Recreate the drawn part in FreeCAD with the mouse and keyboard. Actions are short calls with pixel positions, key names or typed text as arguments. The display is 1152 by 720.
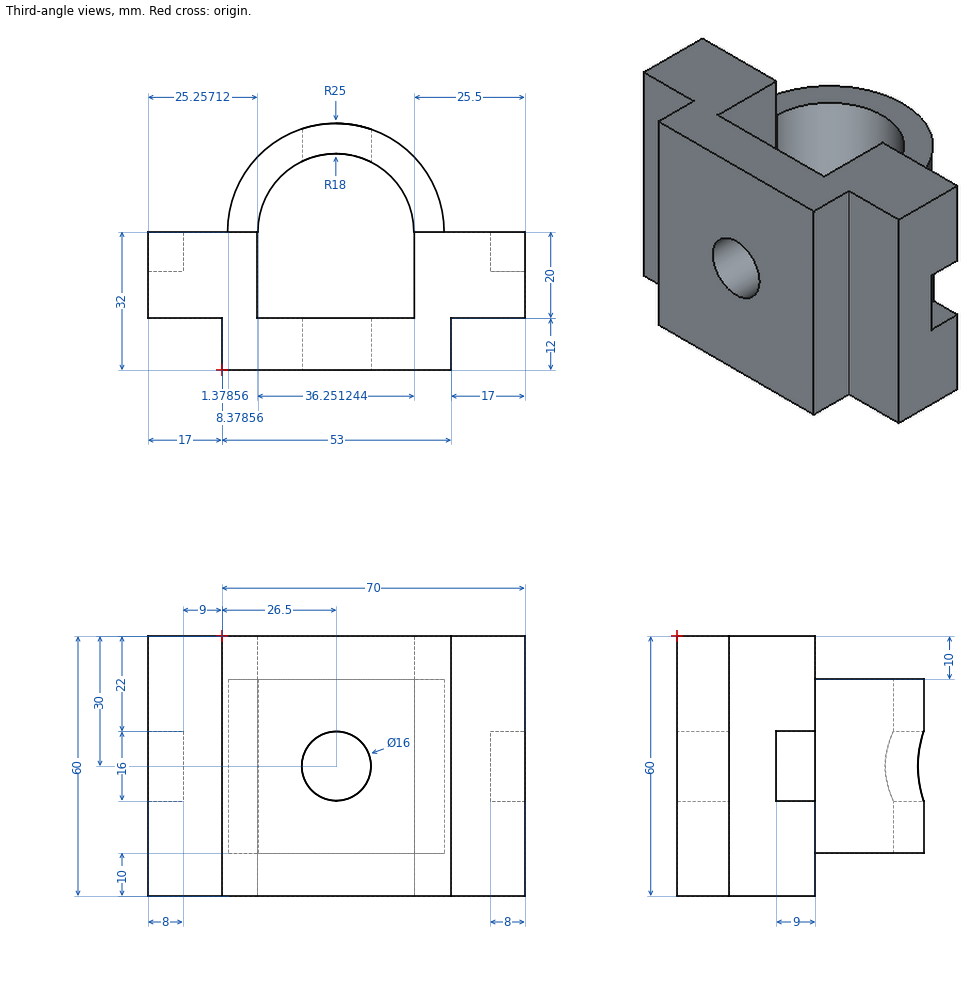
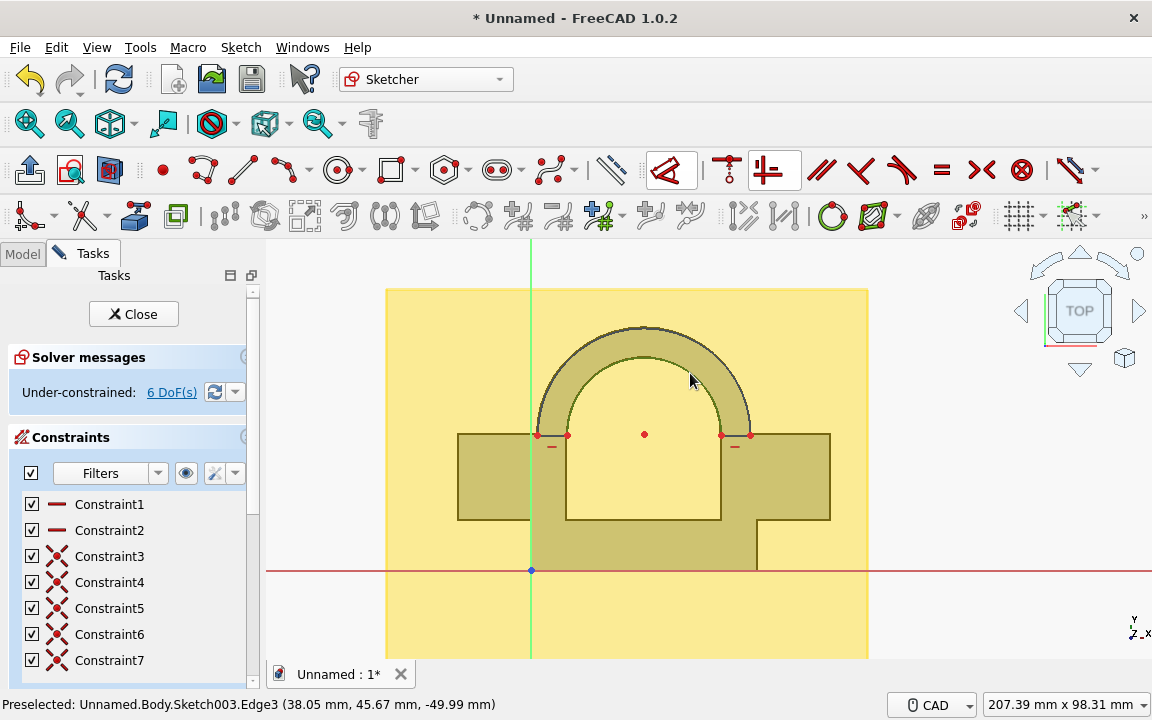
key(k)
key(r)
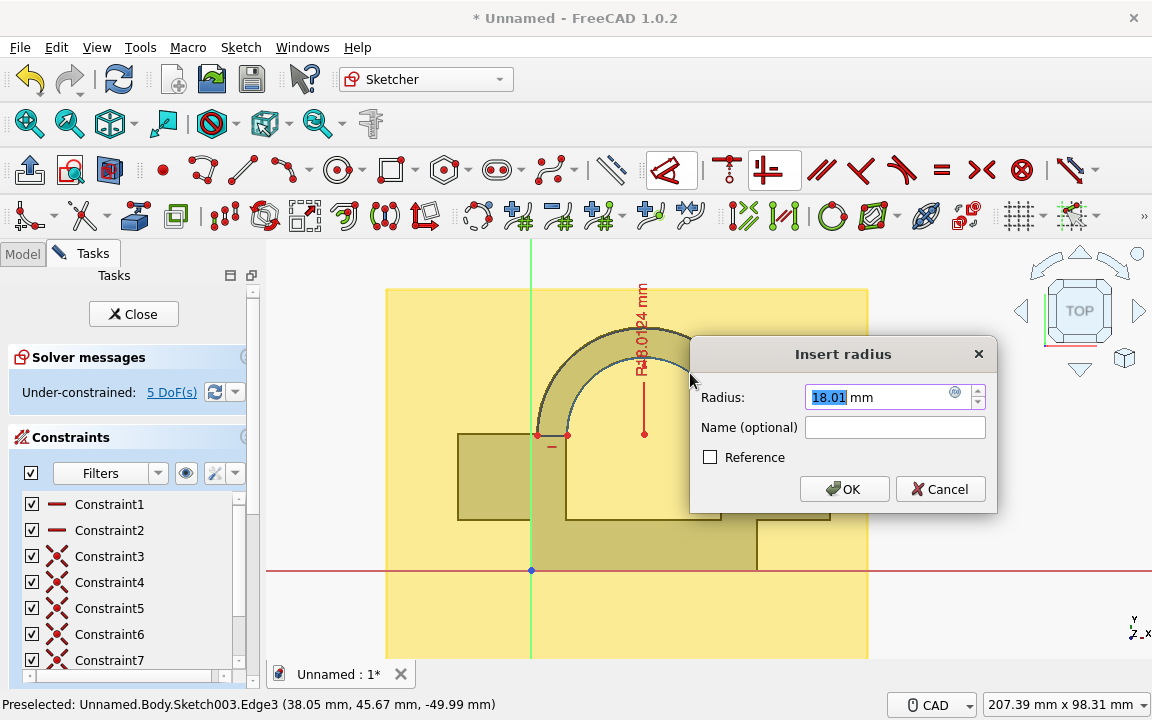
text(18)
key(Return)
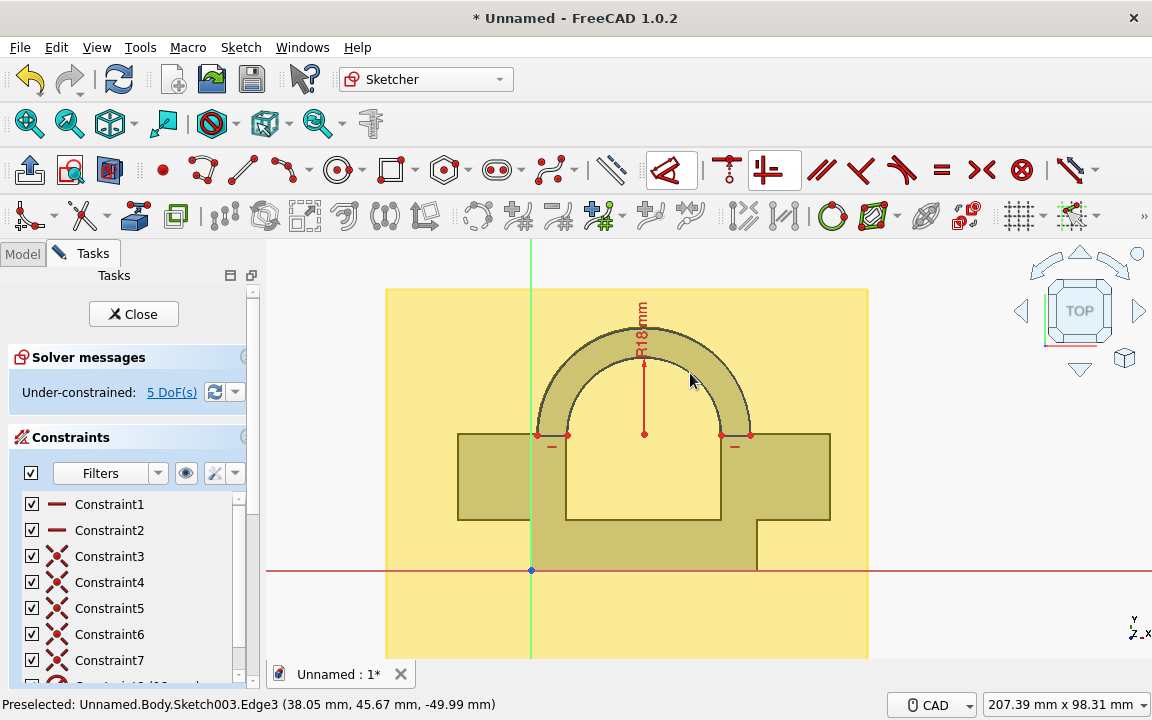
click(707, 349)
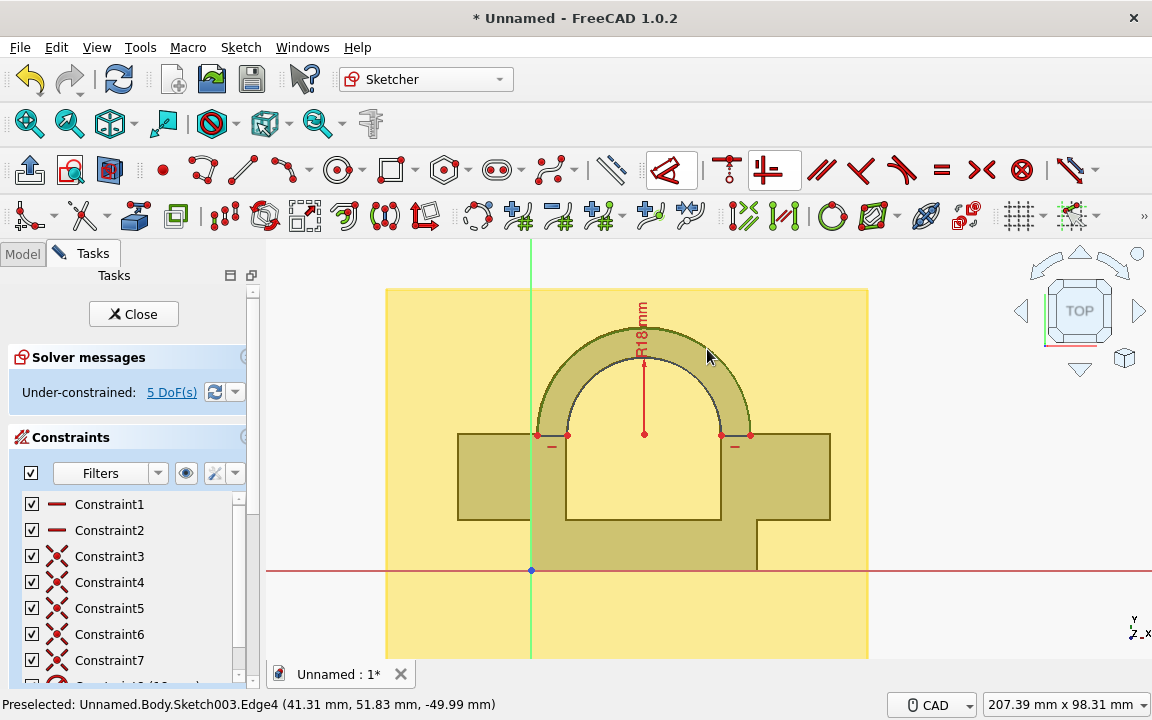
key(k)
key(r)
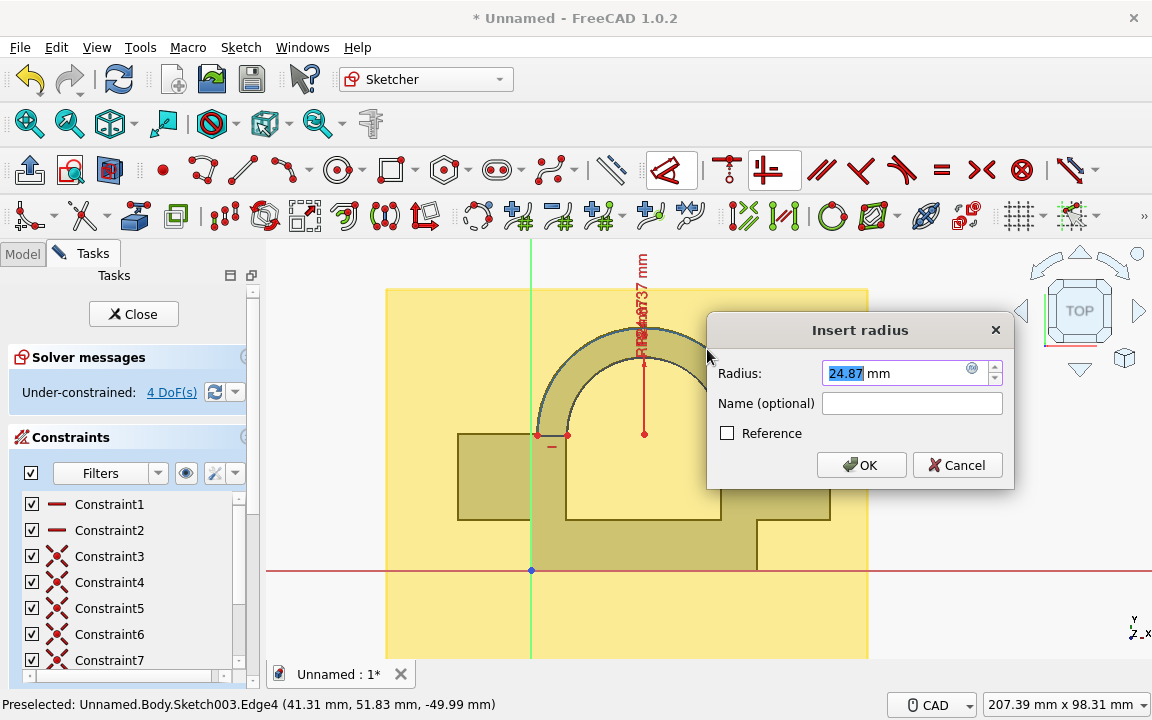
text(25)
key(Return)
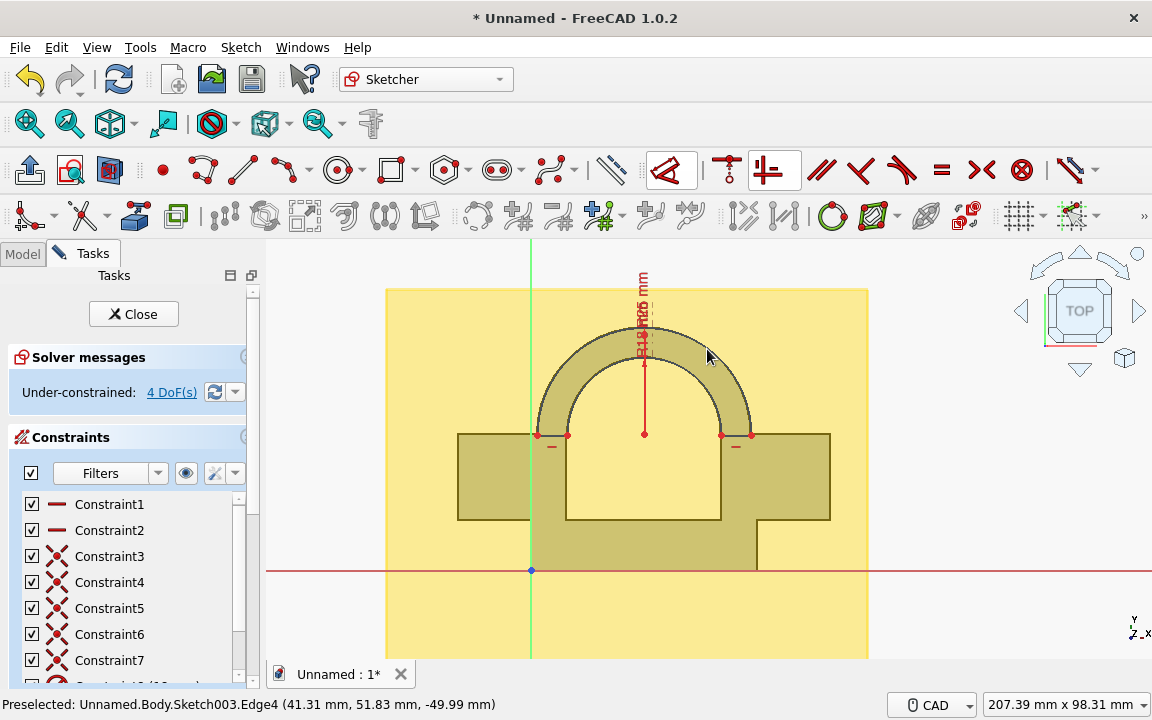
click(751, 436)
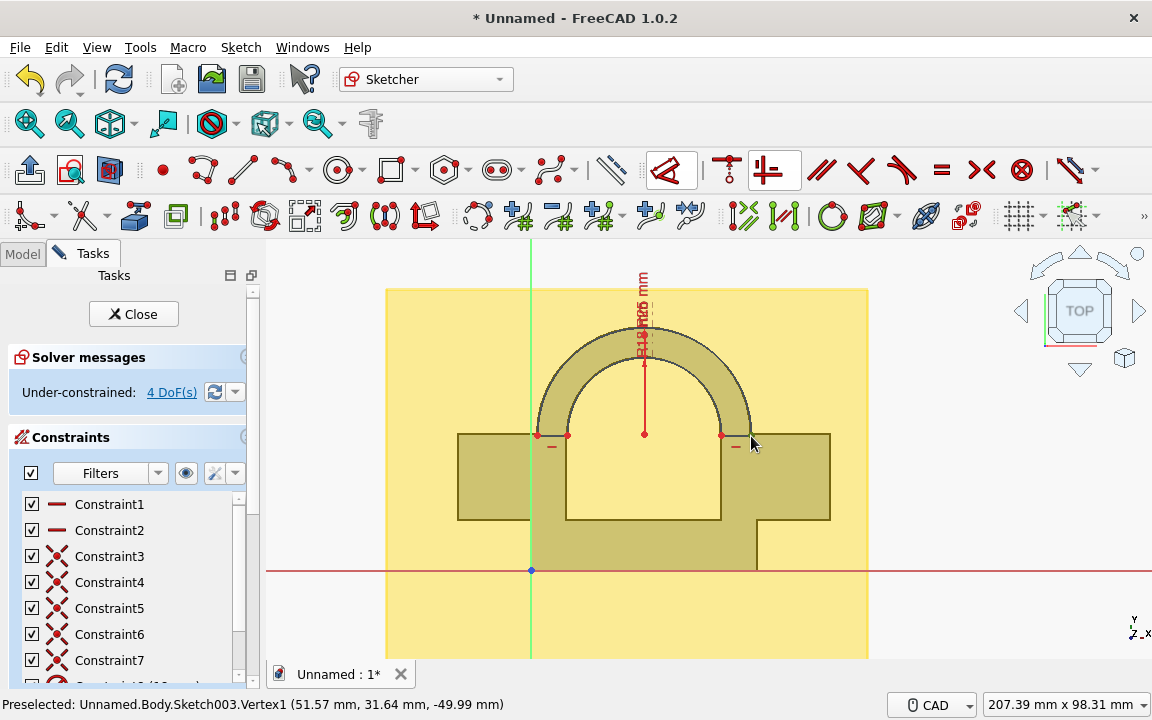
key(i)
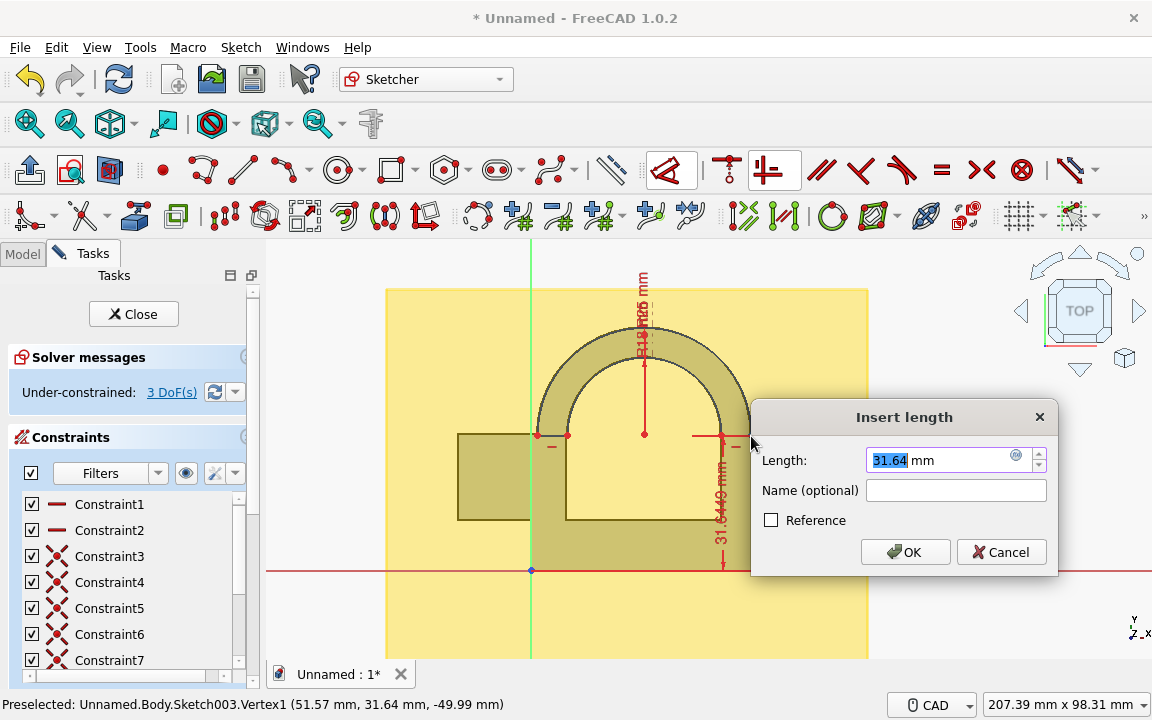
text(32)
key(Return)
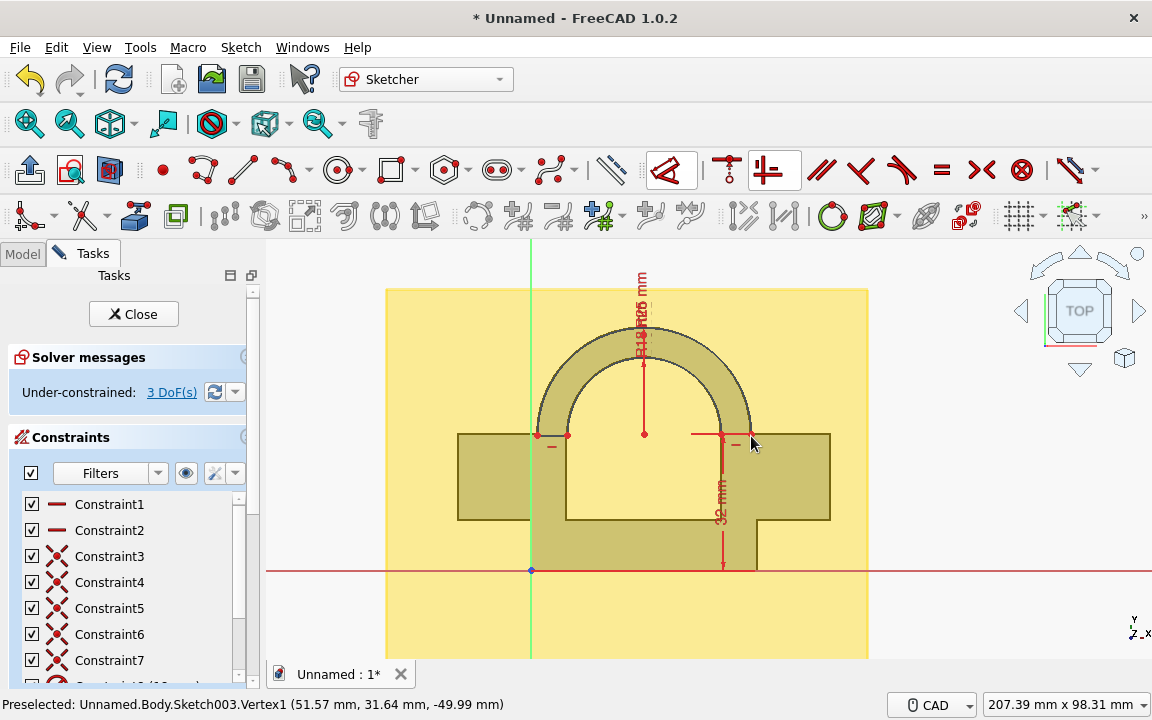
click(568, 436)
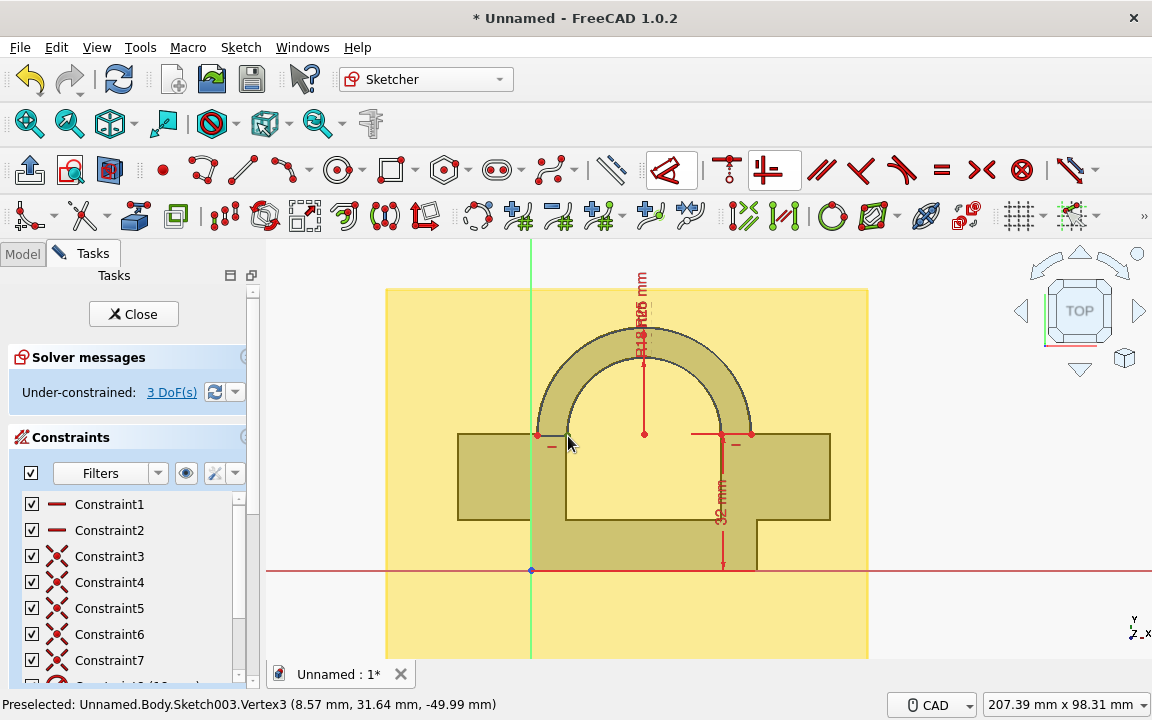
key(i)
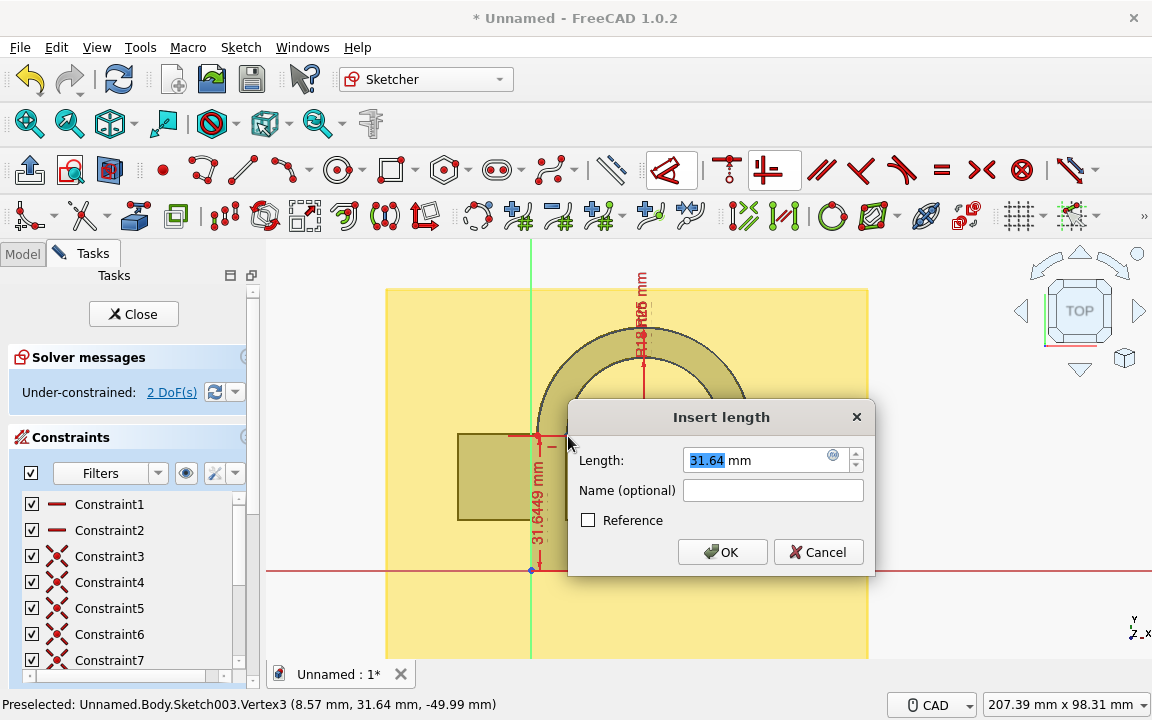
text(32)
key(Return)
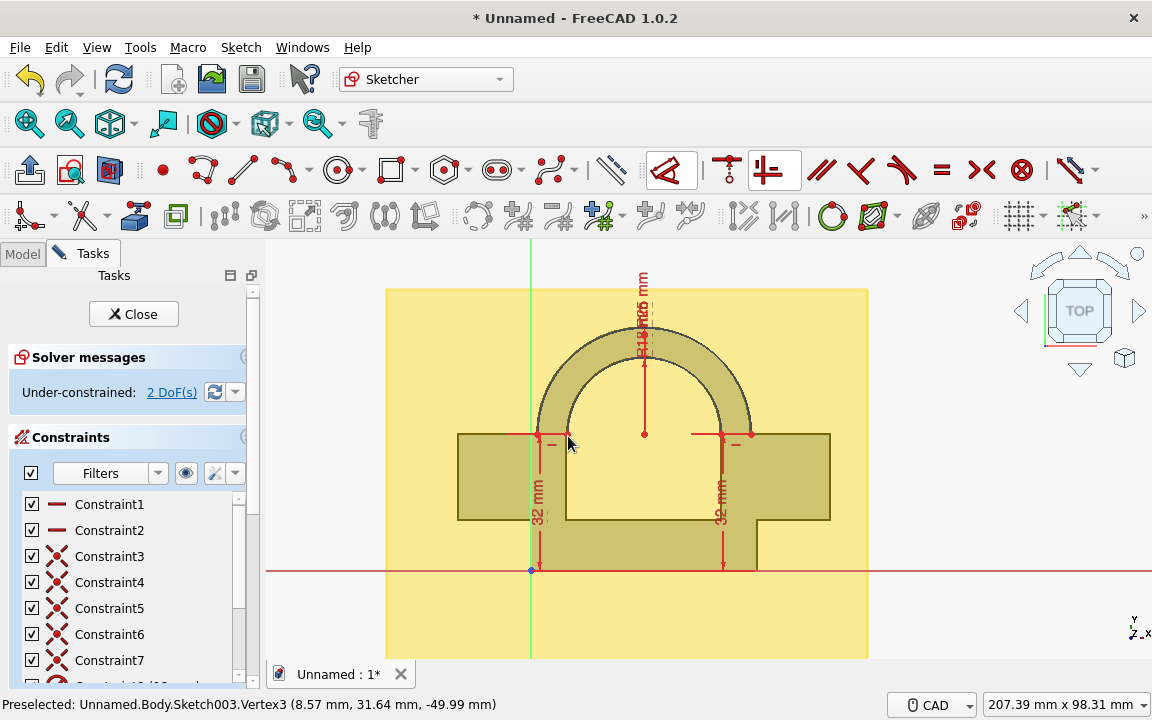
click(645, 435)